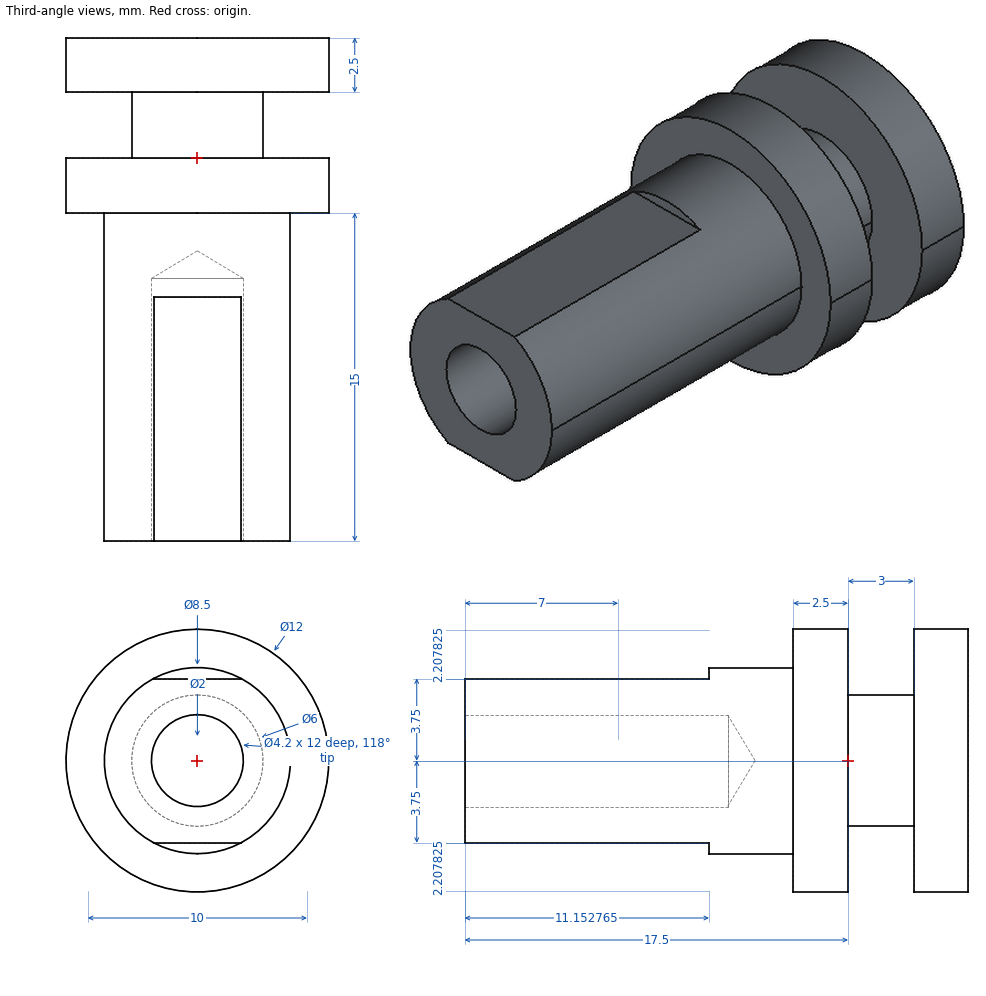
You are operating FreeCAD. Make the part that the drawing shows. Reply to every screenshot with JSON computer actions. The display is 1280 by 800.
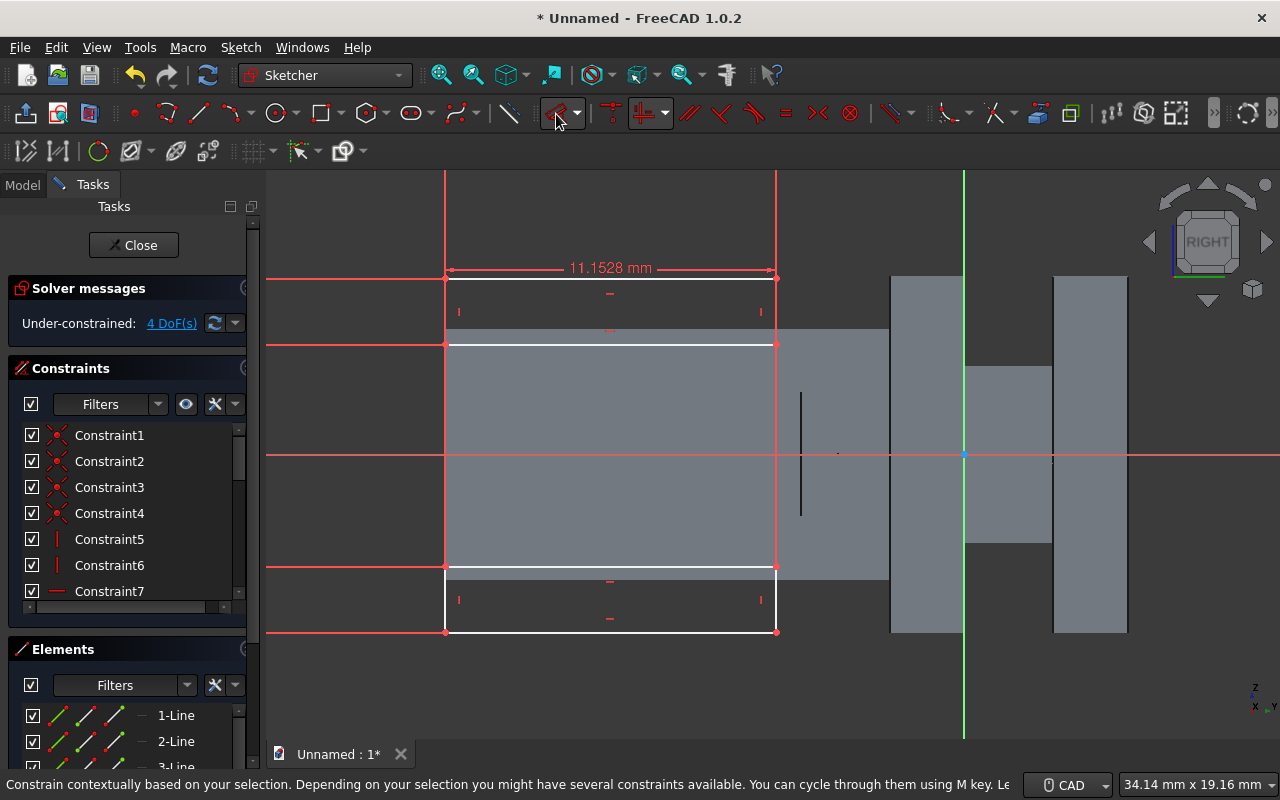
{"action": "left_click", "coordinate": [445, 567]}
{"action": "left_click", "coordinate": [705, 601]}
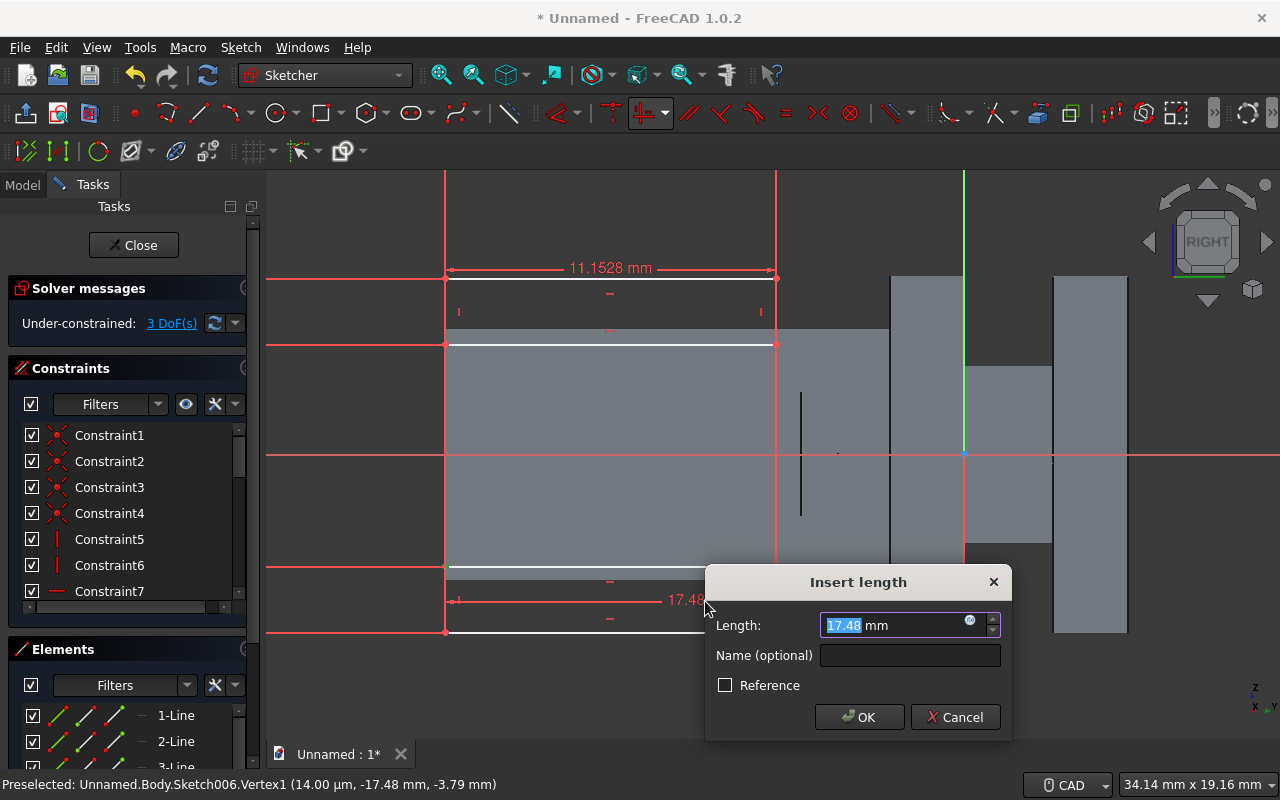
{"action": "type", "text": "17.5"}
{"action": "key", "text": "Return"}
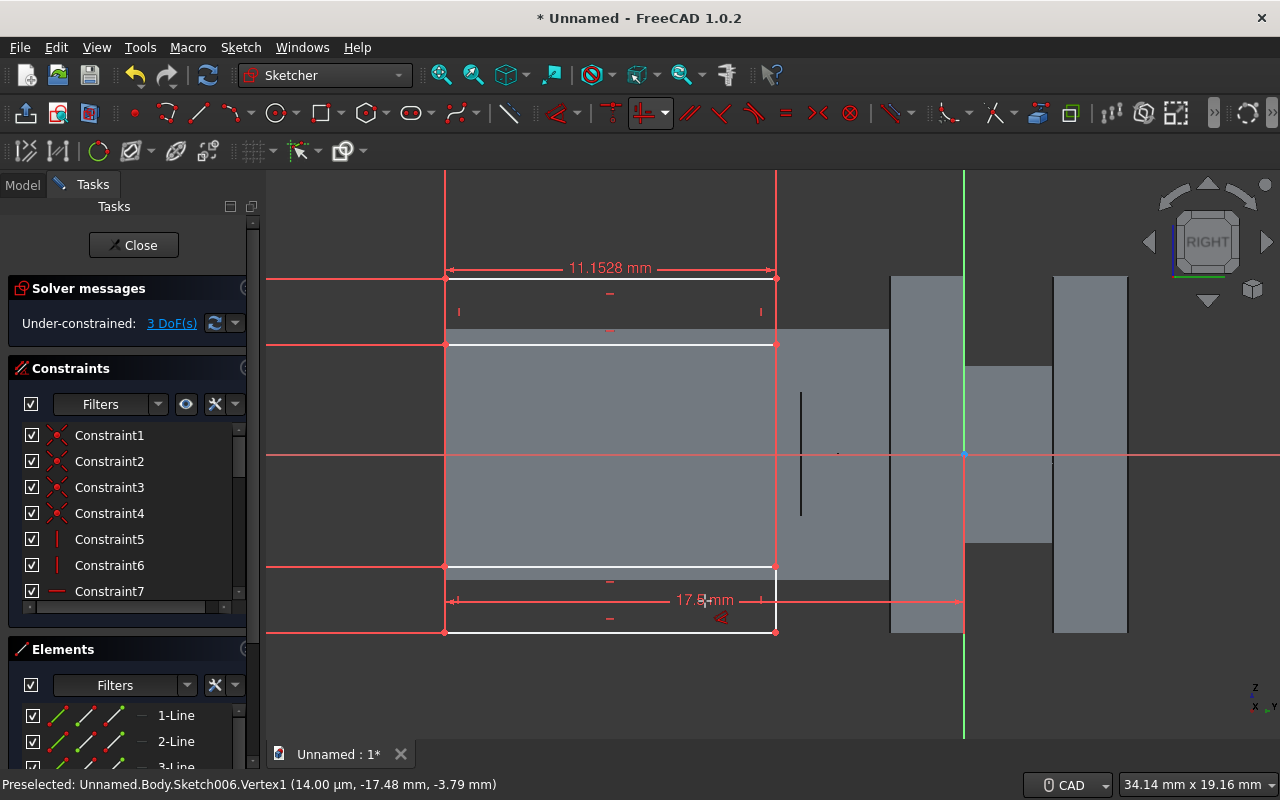
{"action": "left_click", "coordinate": [445, 567]}
{"action": "left_click", "coordinate": [998, 511]}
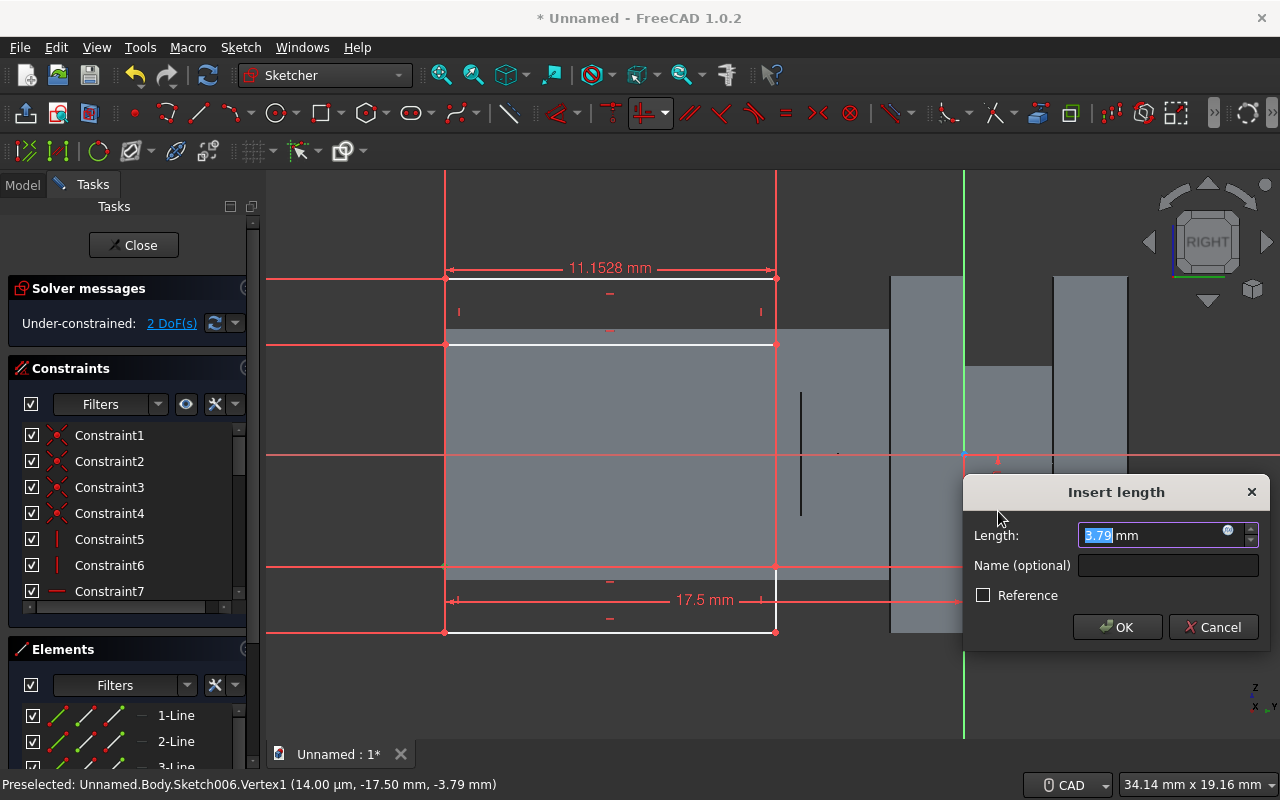
{"action": "type", "text": "3.75"}
{"action": "key", "text": "Return"}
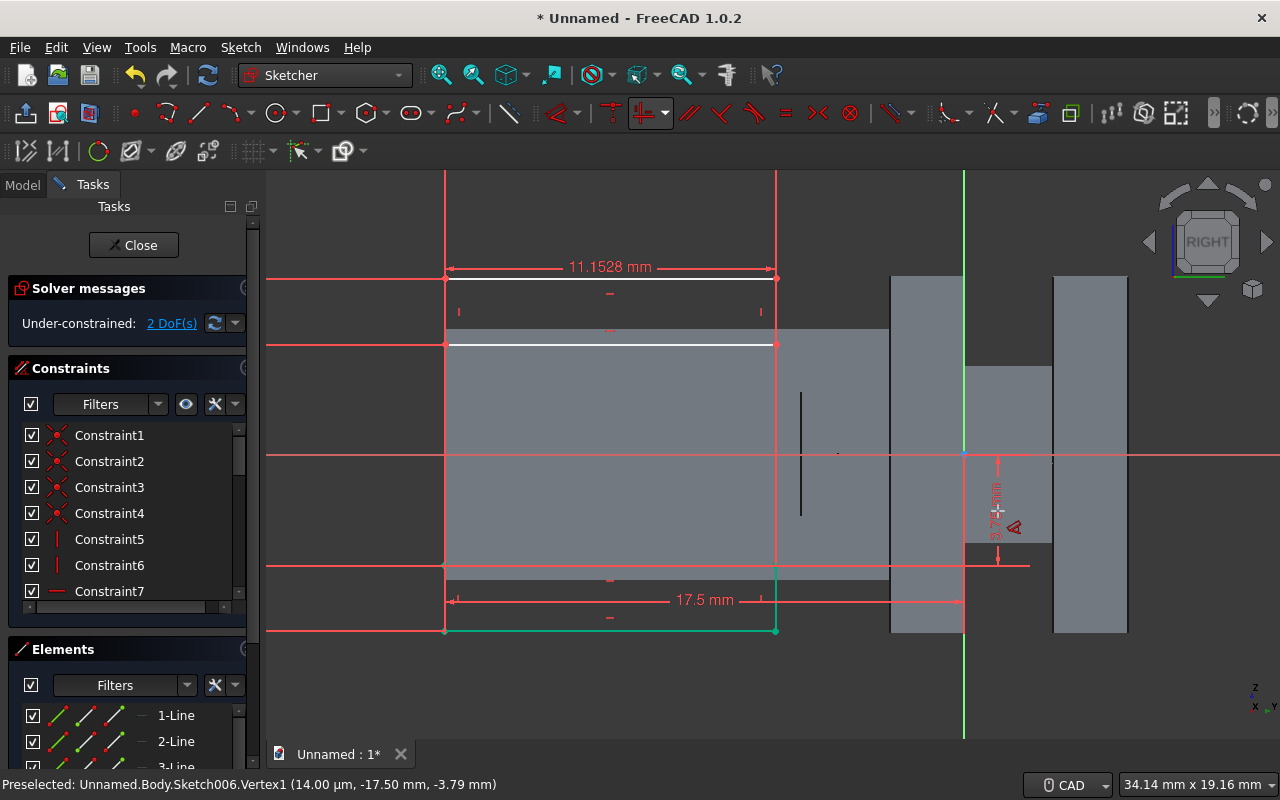
{"action": "left_click", "coordinate": [445, 279]}
{"action": "left_click", "coordinate": [705, 245]}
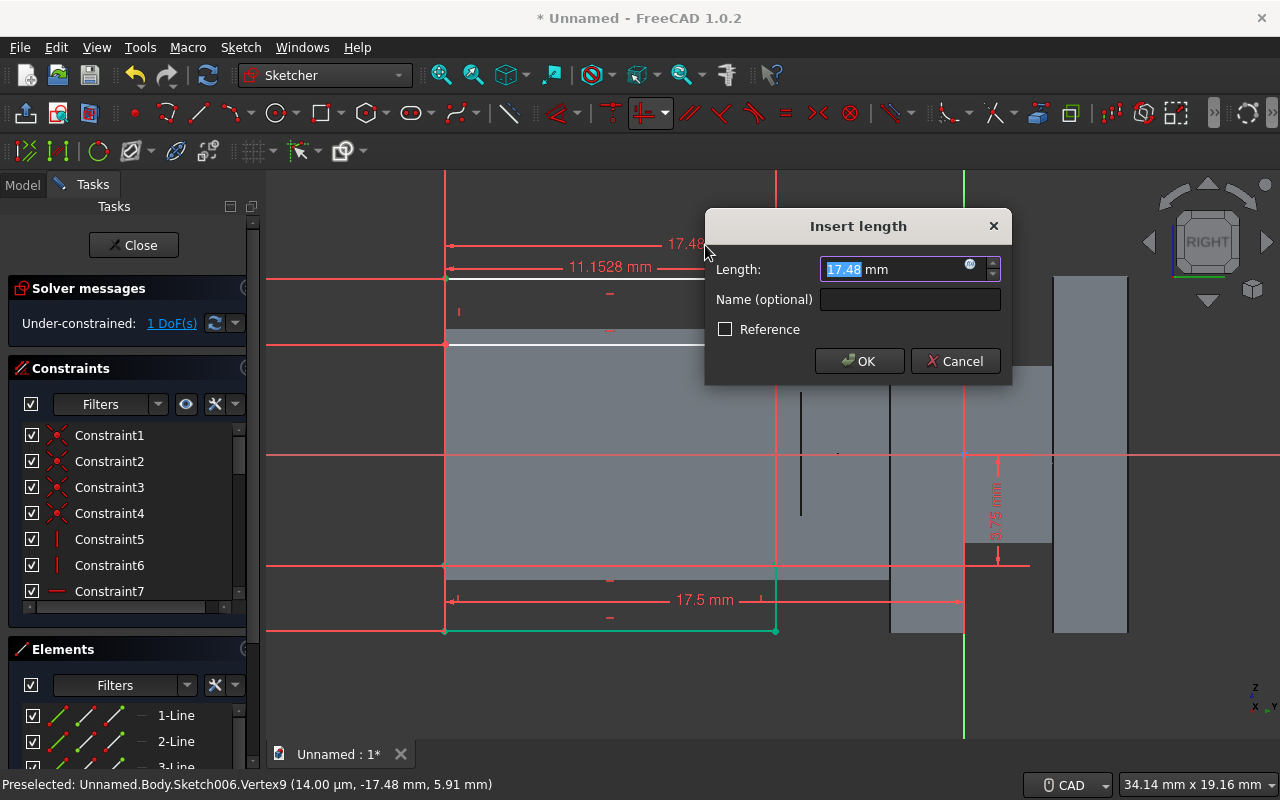
{"action": "type", "text": "17.5"}
{"action": "key", "text": "Return"}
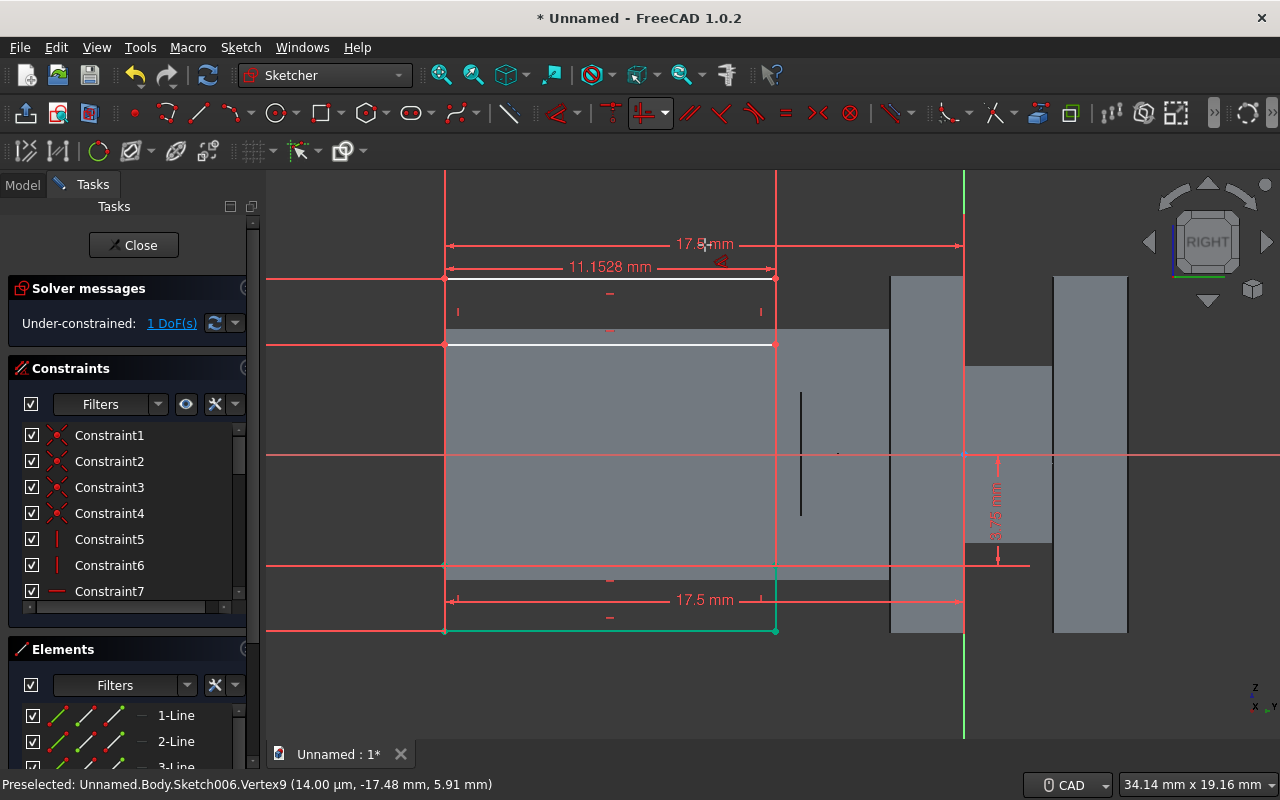
{"action": "left_click", "coordinate": [445, 345]}
{"action": "left_click", "coordinate": [998, 400]}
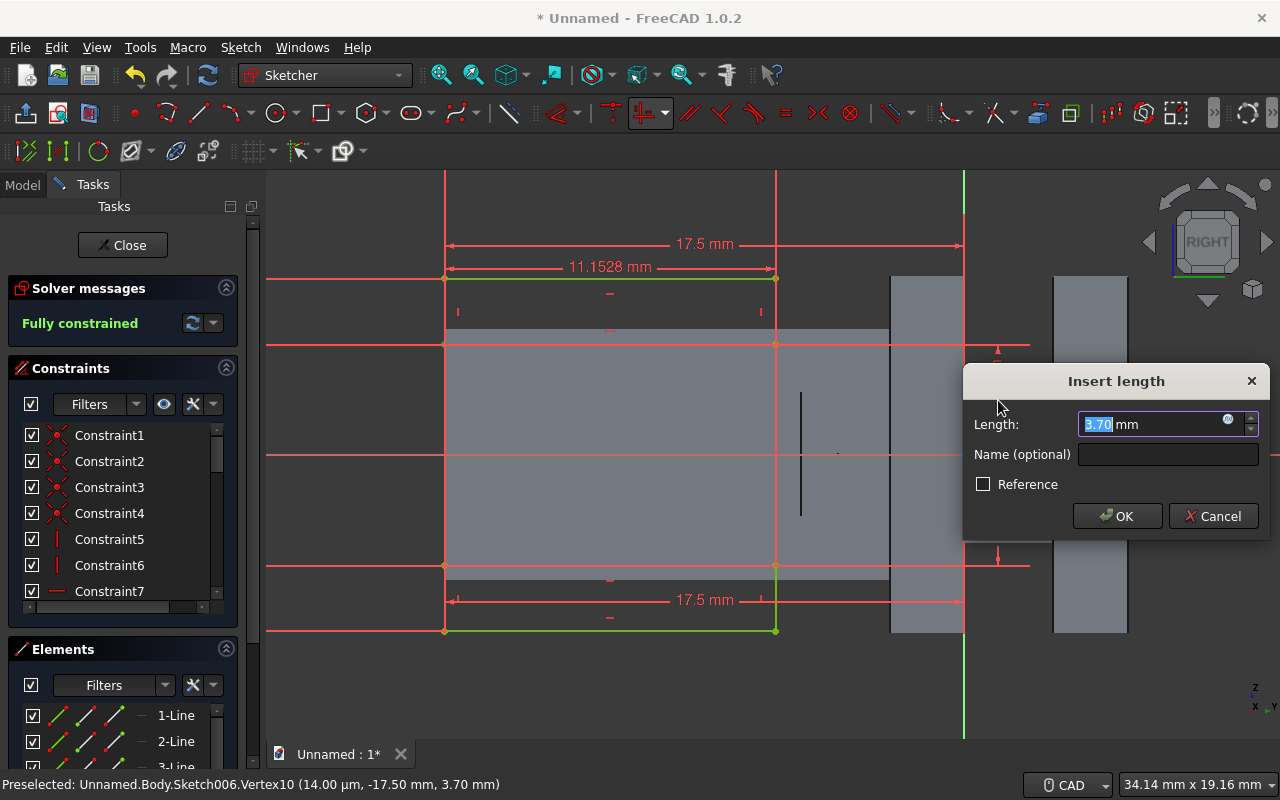
{"action": "type", "text": "3.75"}
{"action": "key", "text": "Return"}
{"action": "key", "text": "Escape"}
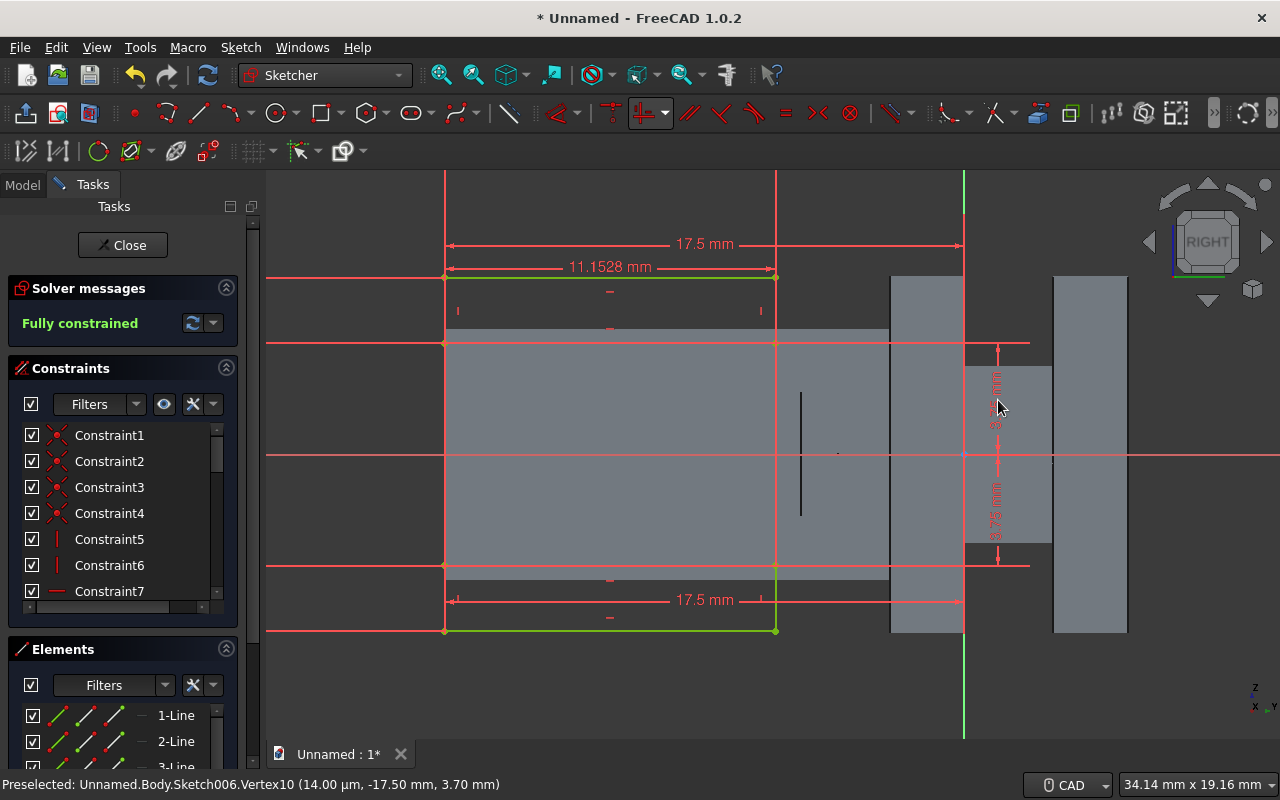
{"action": "left_click", "coordinate": [123, 245]}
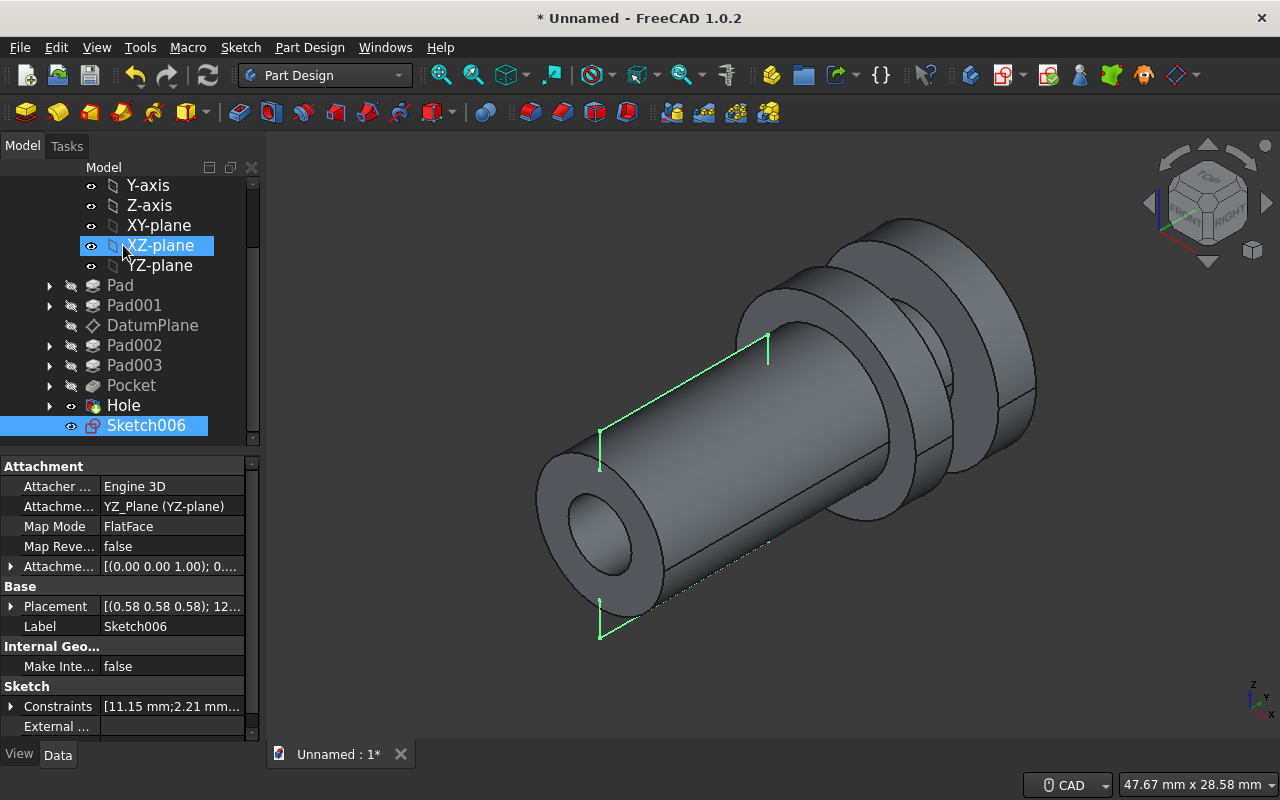
{"action": "left_click", "coordinate": [240, 112]}